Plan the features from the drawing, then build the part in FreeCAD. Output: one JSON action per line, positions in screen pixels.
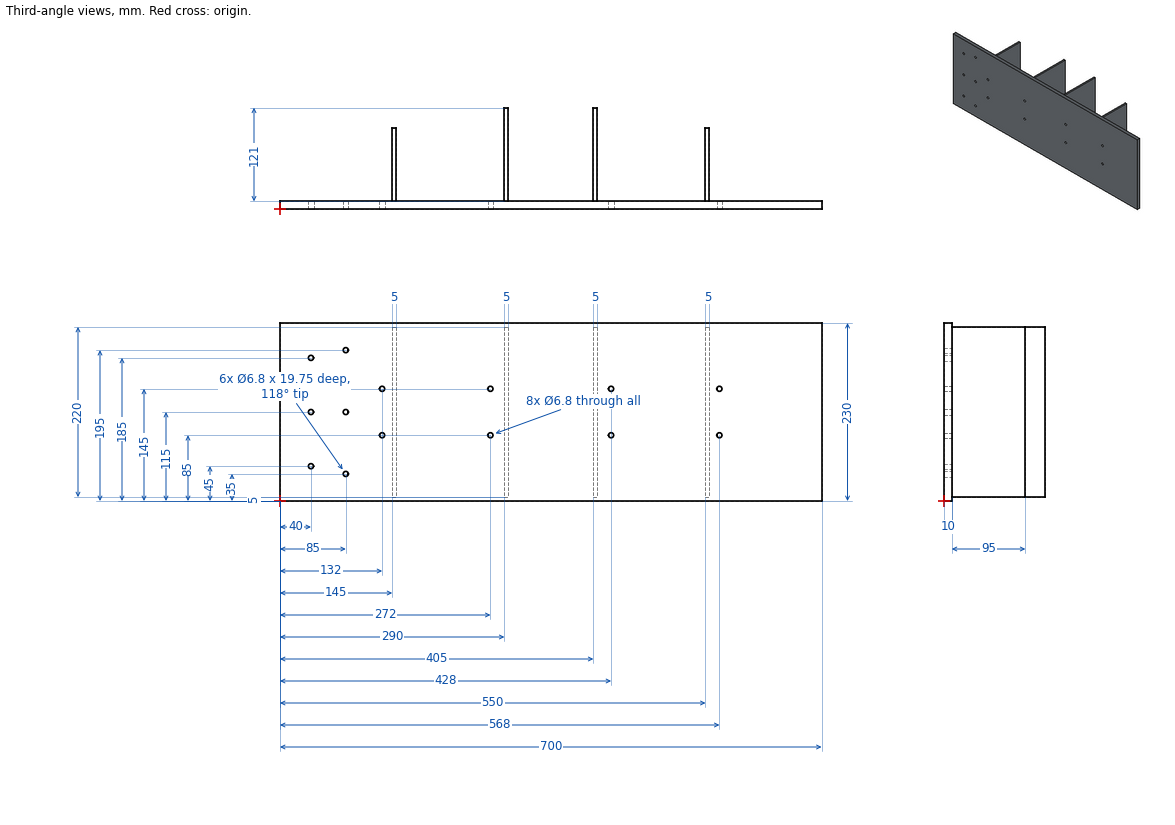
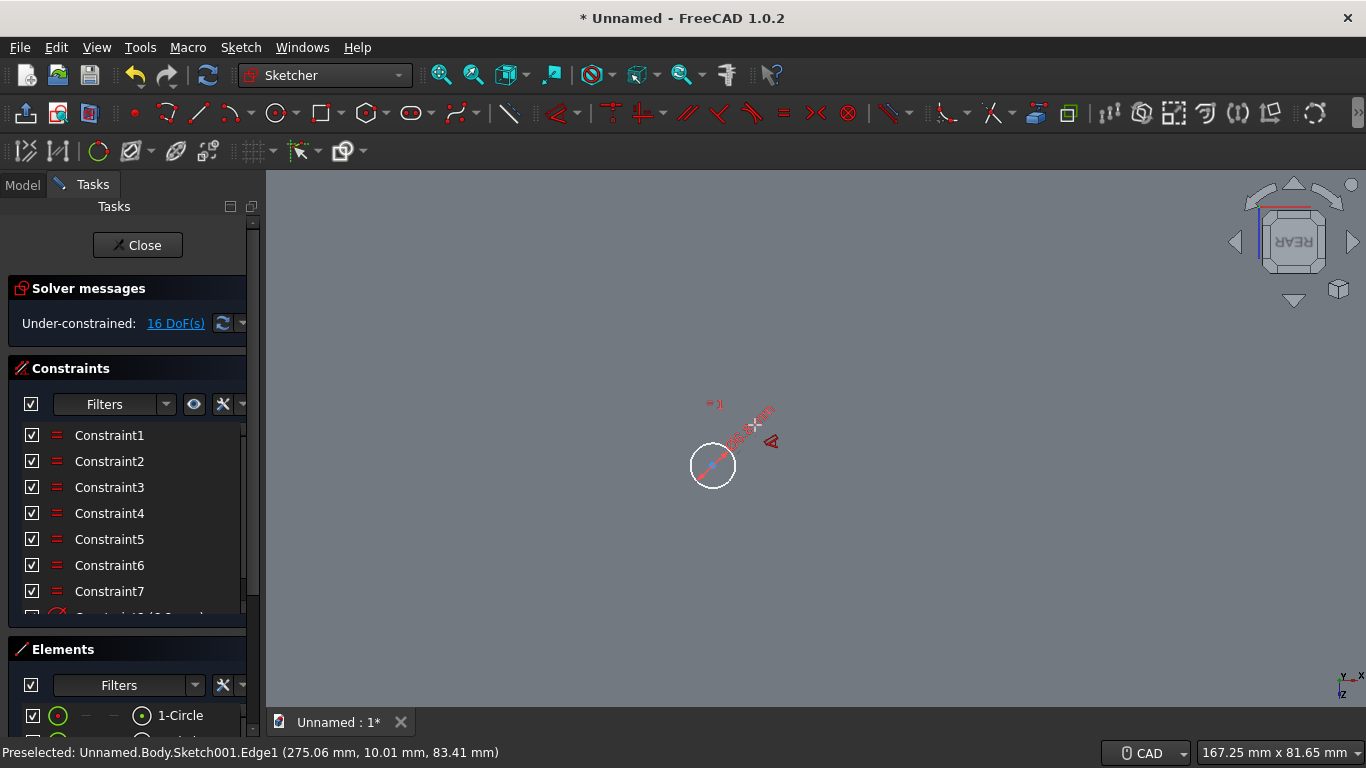
{"action": "scroll", "coordinate": [736, 448], "scroll_direction": "down", "scroll_amount": 9}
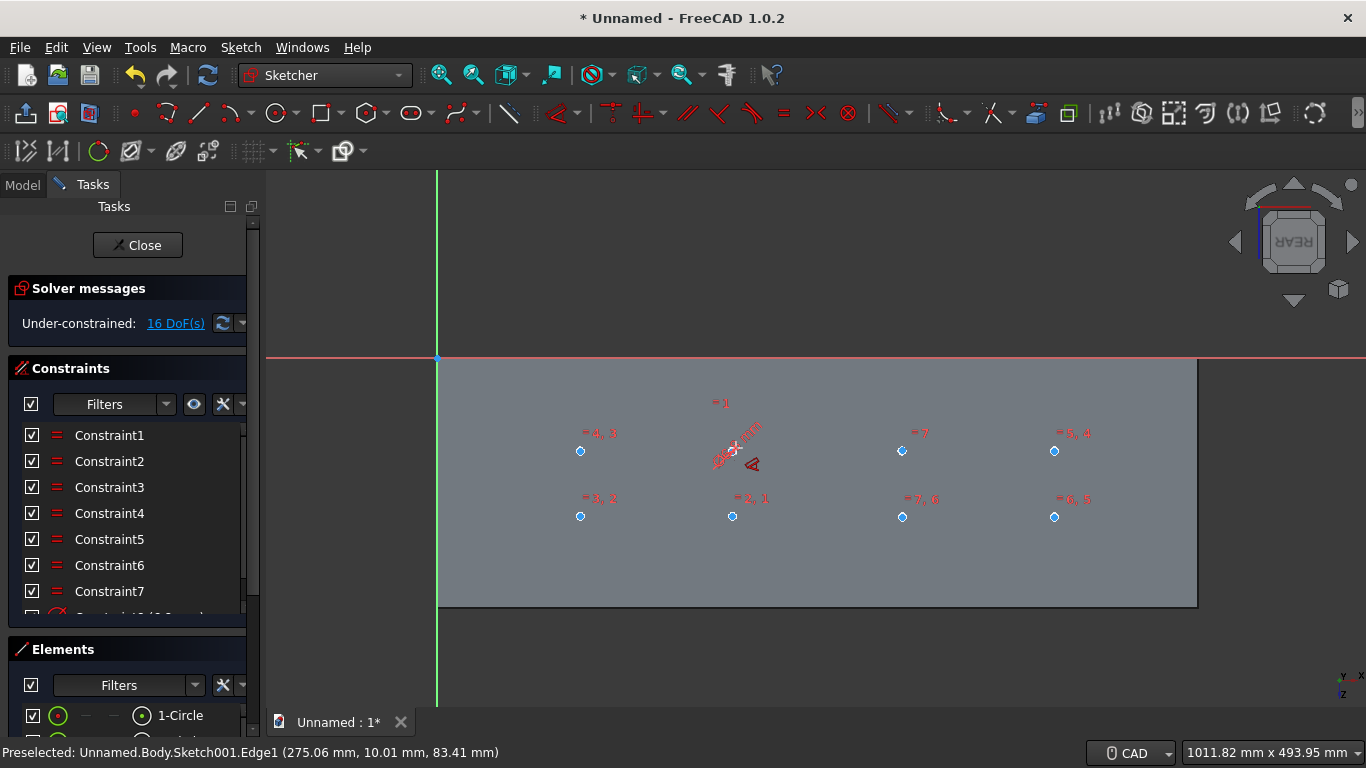
{"action": "left_click", "coordinate": [733, 451]}
{"action": "left_click", "coordinate": [403, 405]}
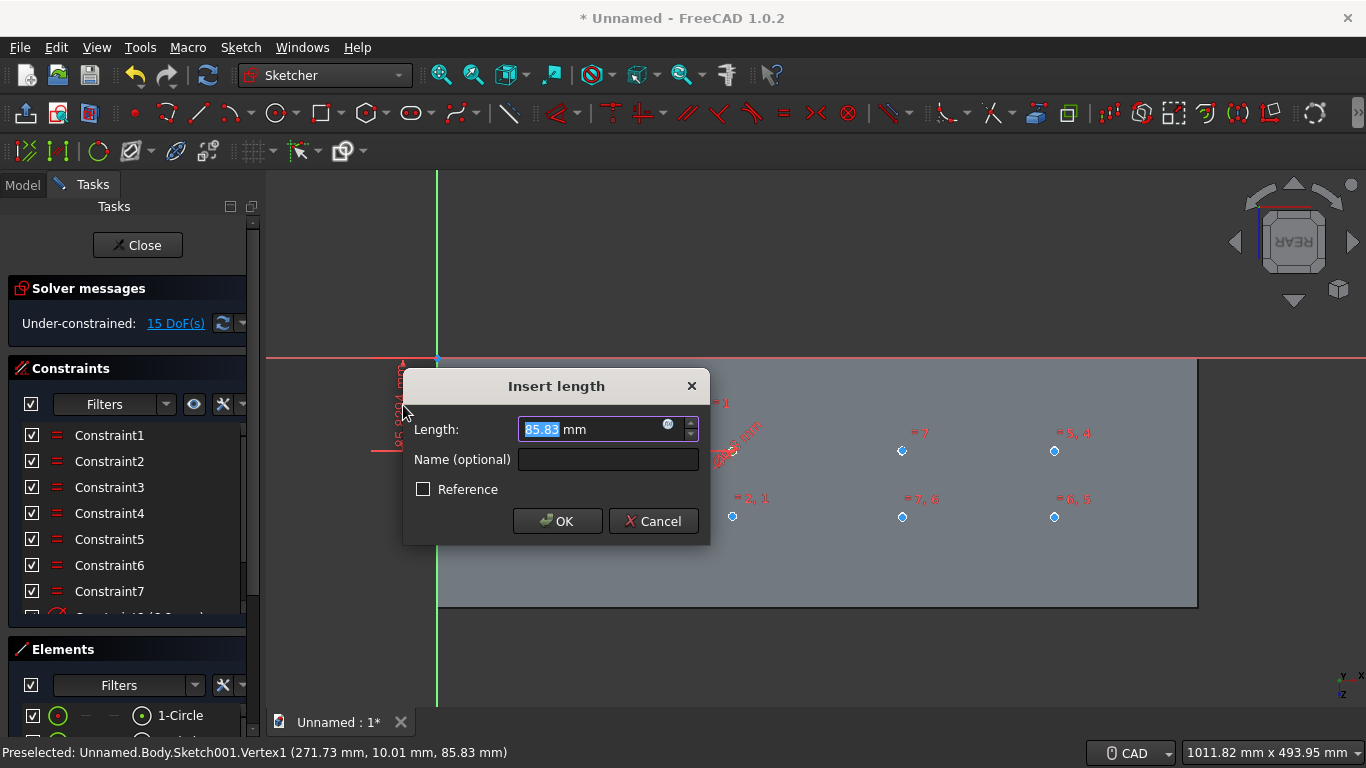
{"action": "type", "text": "85"}
{"action": "key", "text": "Return"}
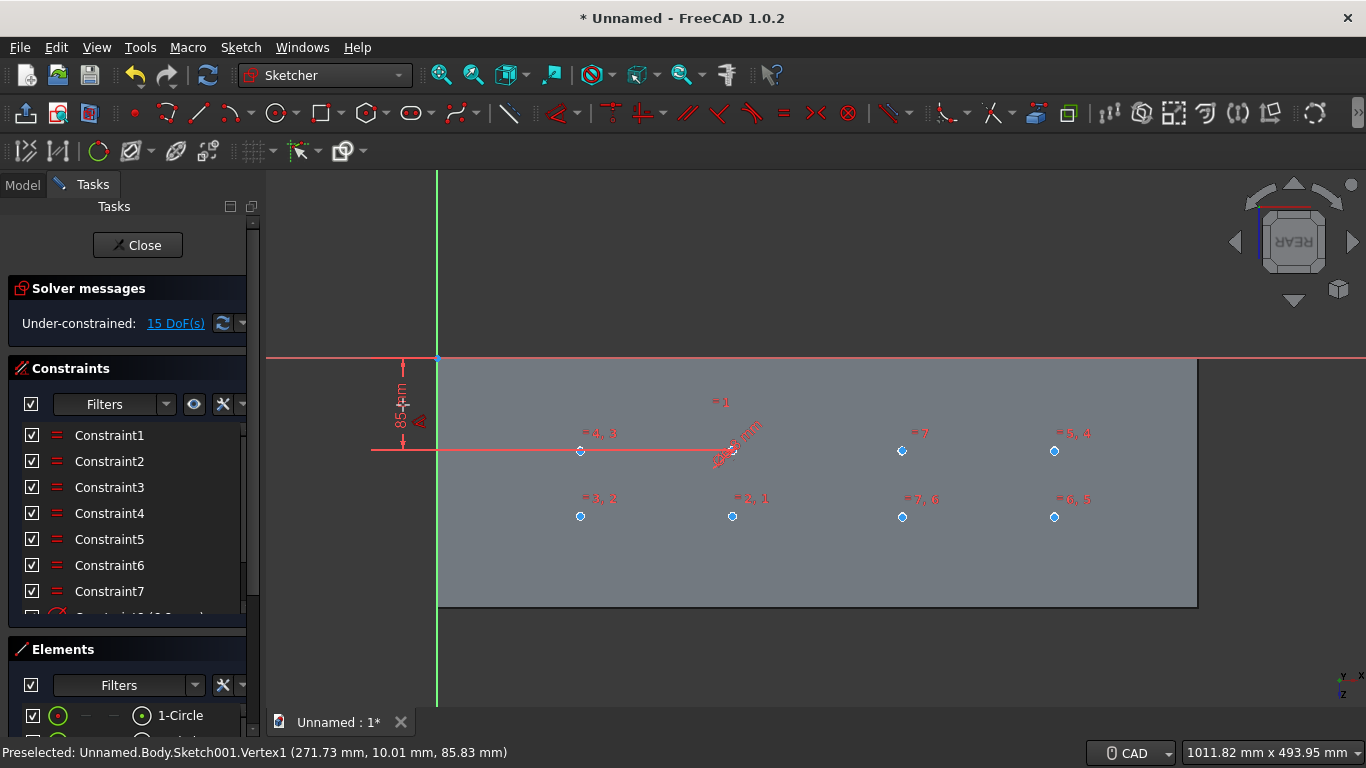
{"action": "left_click", "coordinate": [580, 451]}
{"action": "left_click", "coordinate": [403, 383]}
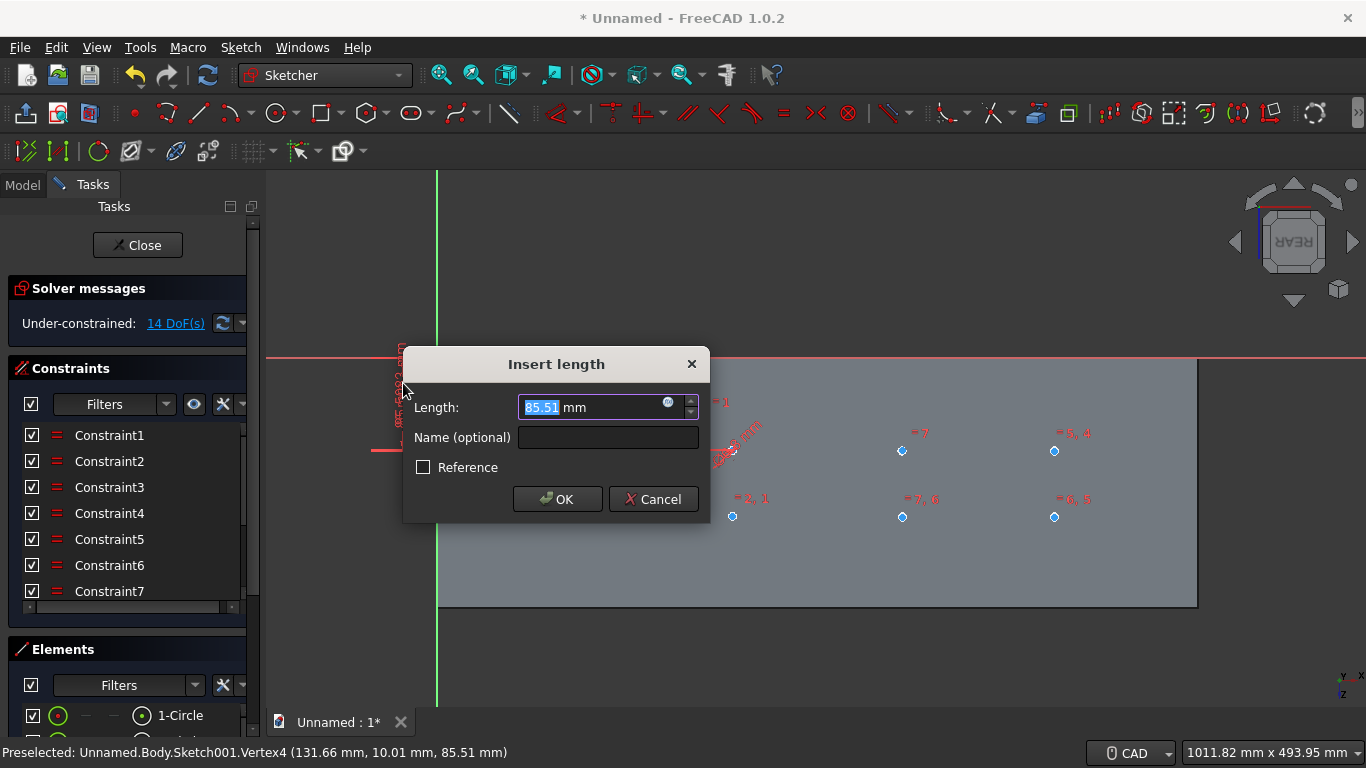
{"action": "type", "text": "85"}
{"action": "key", "text": "Return"}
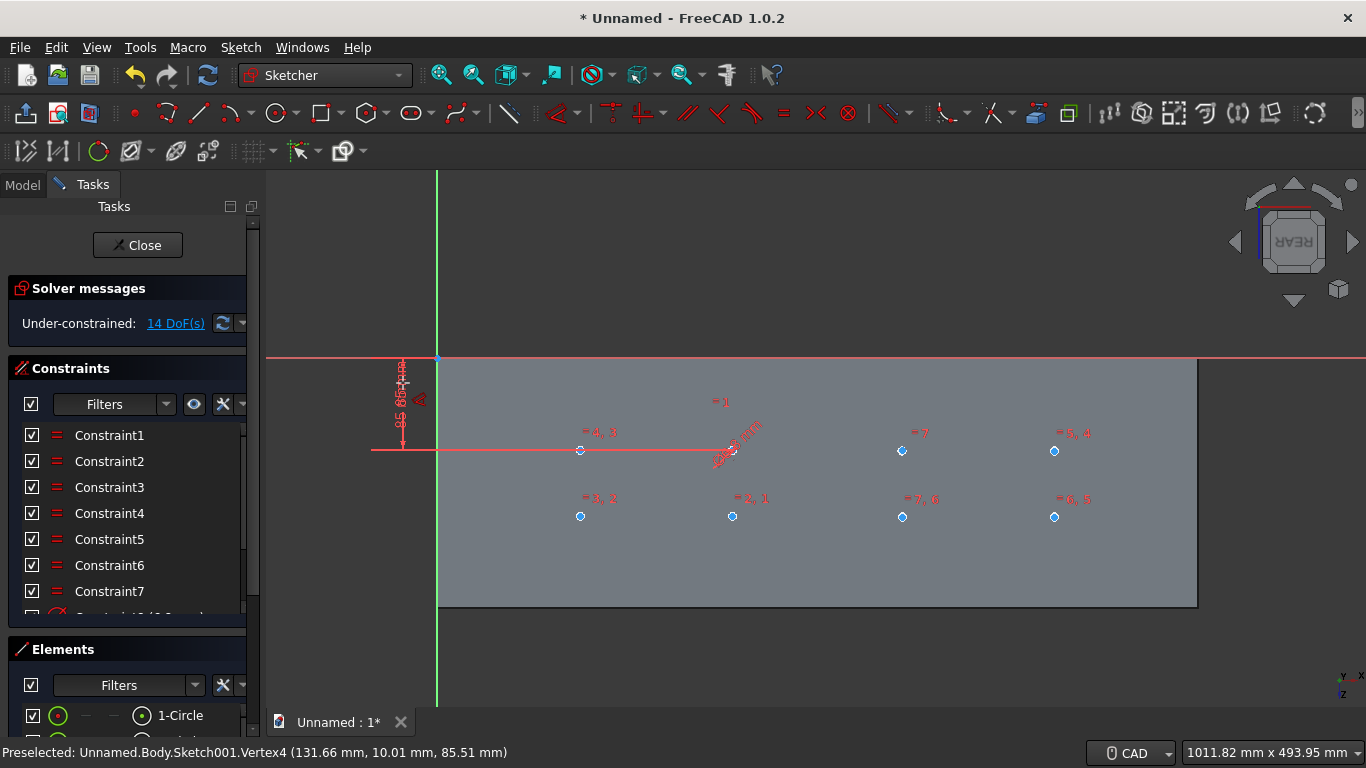
{"action": "left_click", "coordinate": [1054, 451]}
{"action": "left_click", "coordinate": [403, 426]}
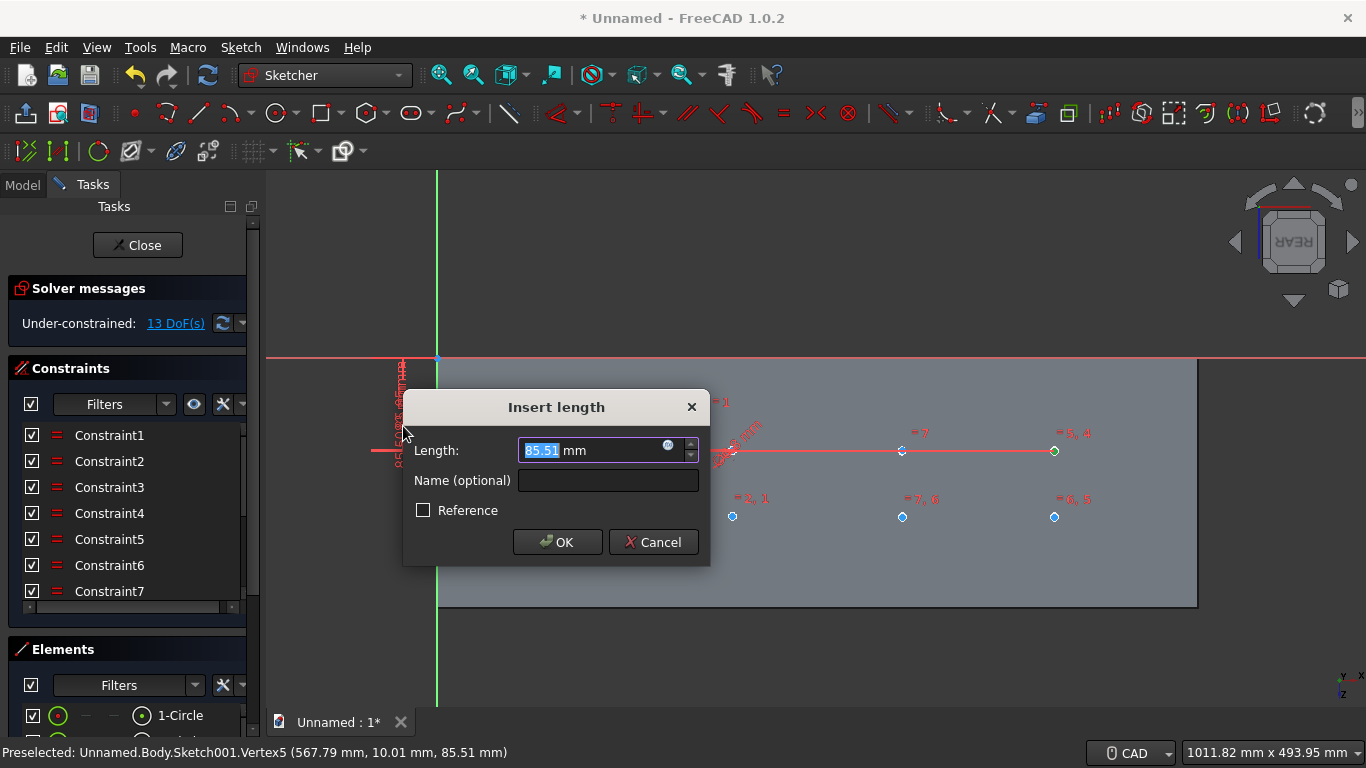
{"action": "type", "text": "85"}
{"action": "key", "text": "Return"}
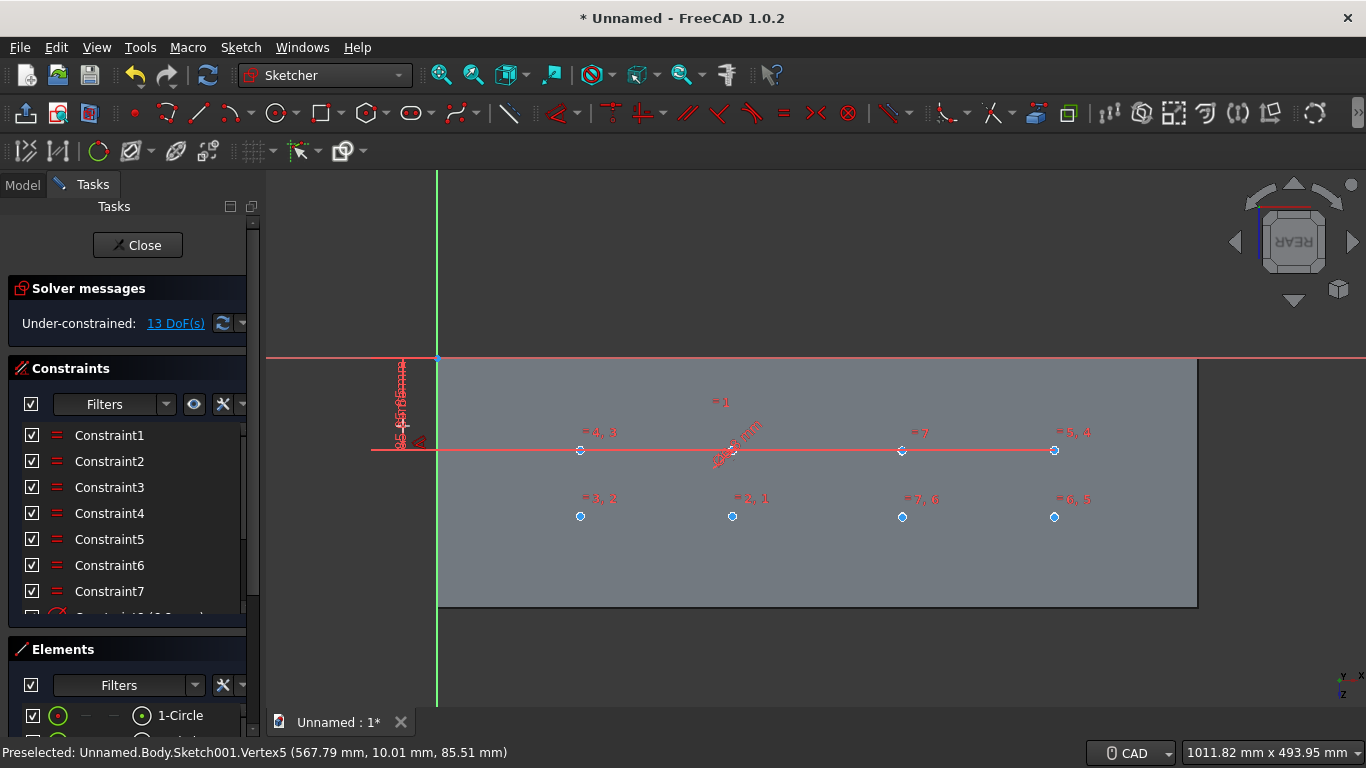
{"action": "left_click", "coordinate": [902, 451]}
{"action": "left_click", "coordinate": [936, 405]}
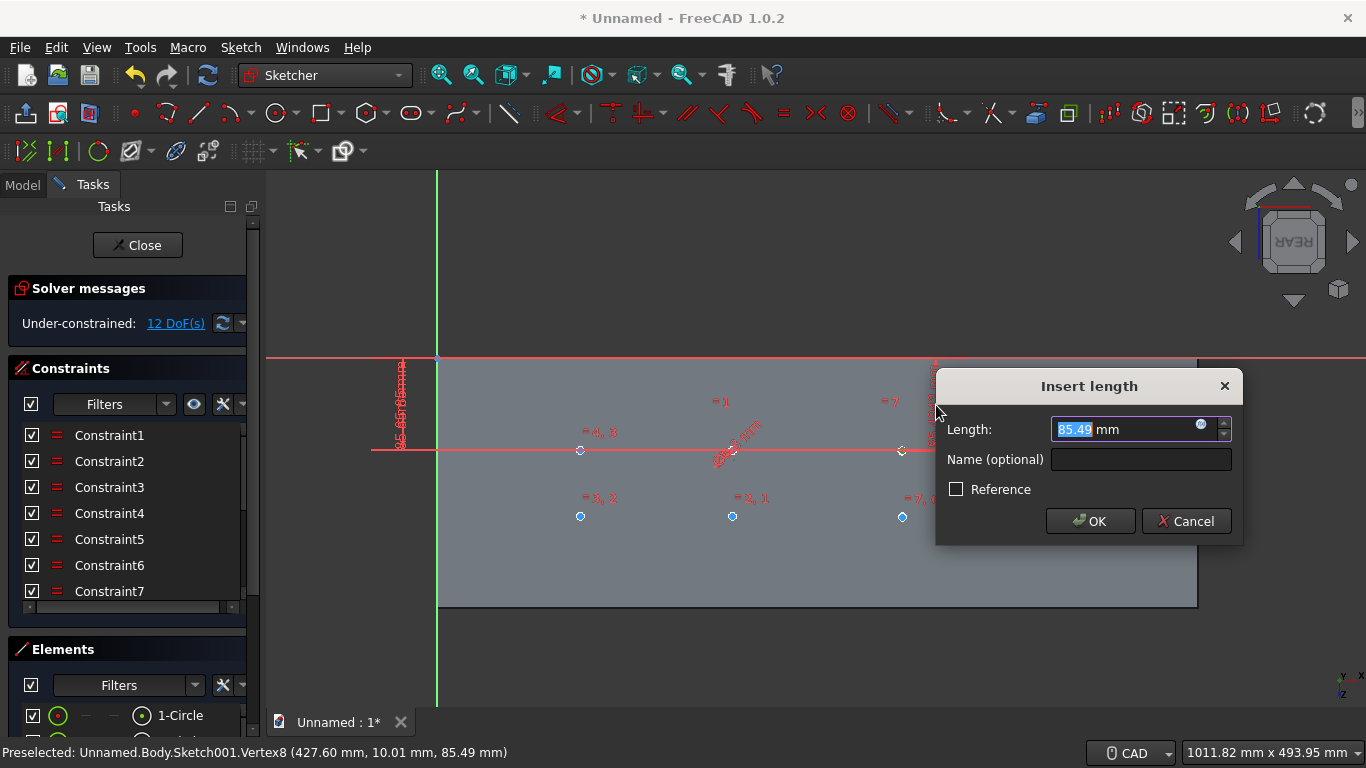
{"action": "type", "text": "85"}
{"action": "key", "text": "Return"}